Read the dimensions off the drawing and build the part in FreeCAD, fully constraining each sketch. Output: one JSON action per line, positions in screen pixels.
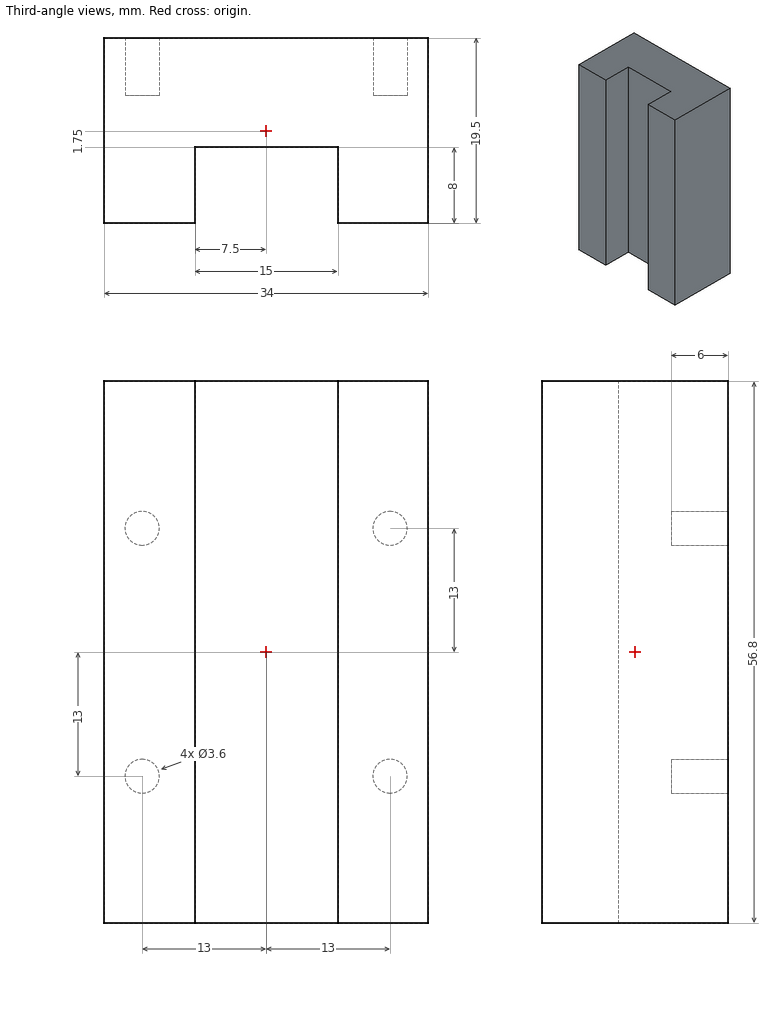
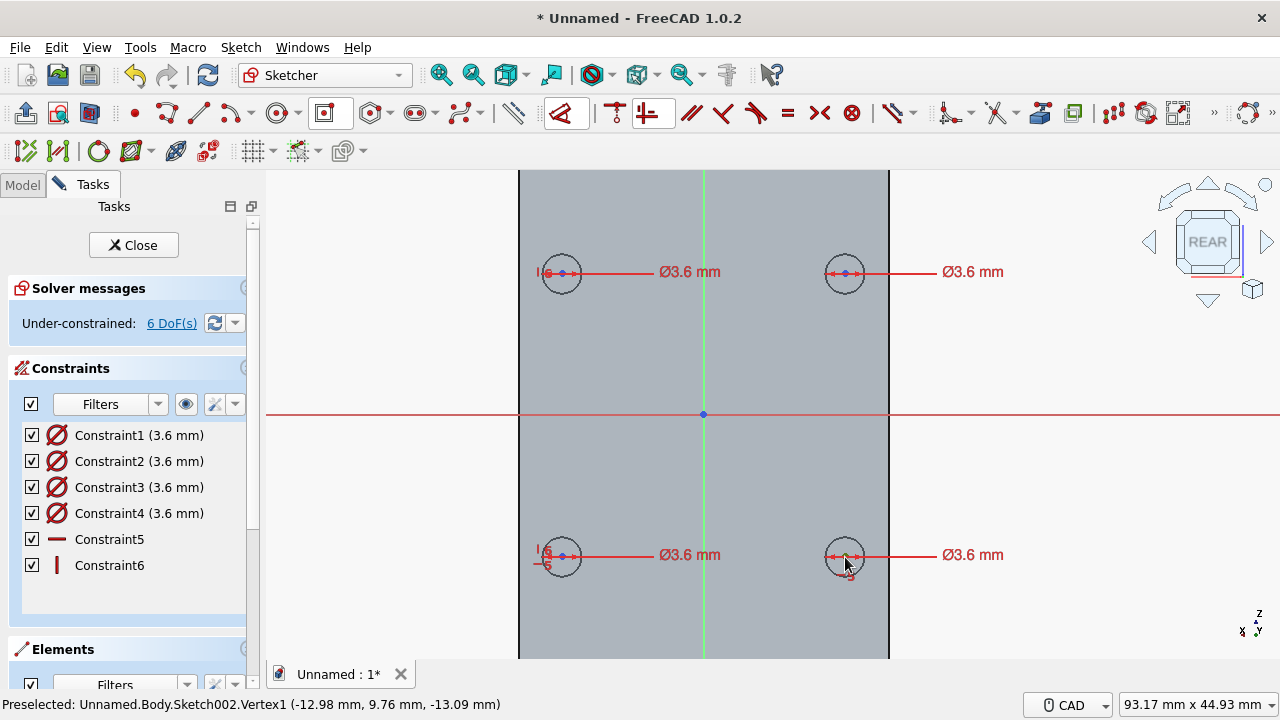
{"action": "left_click", "coordinate": [845, 274]}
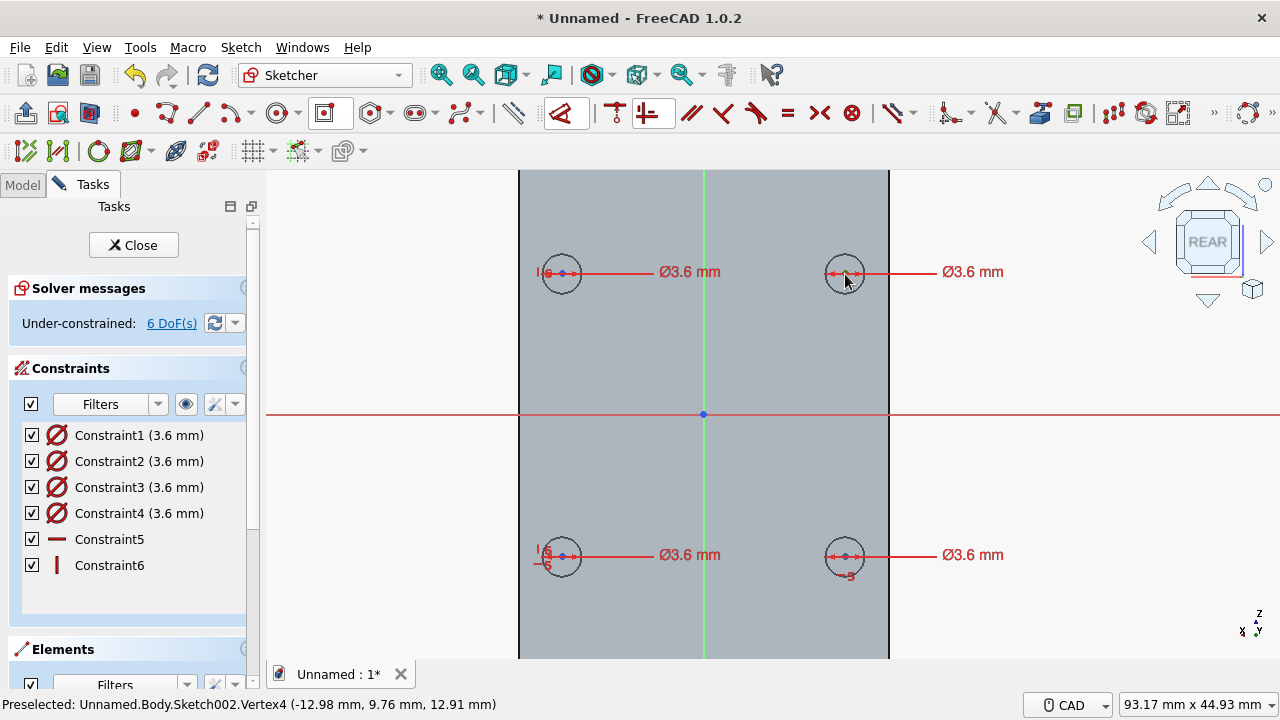
{"action": "key", "text": "v"}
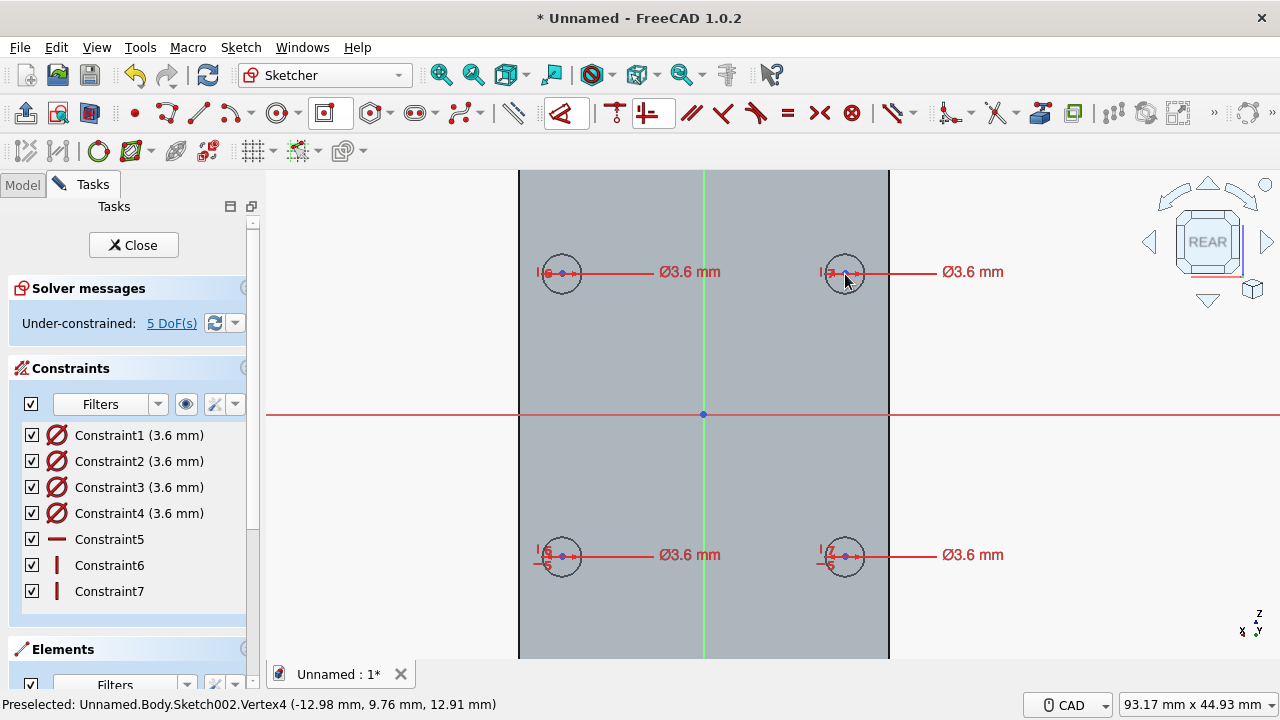
{"action": "left_click", "coordinate": [562, 274]}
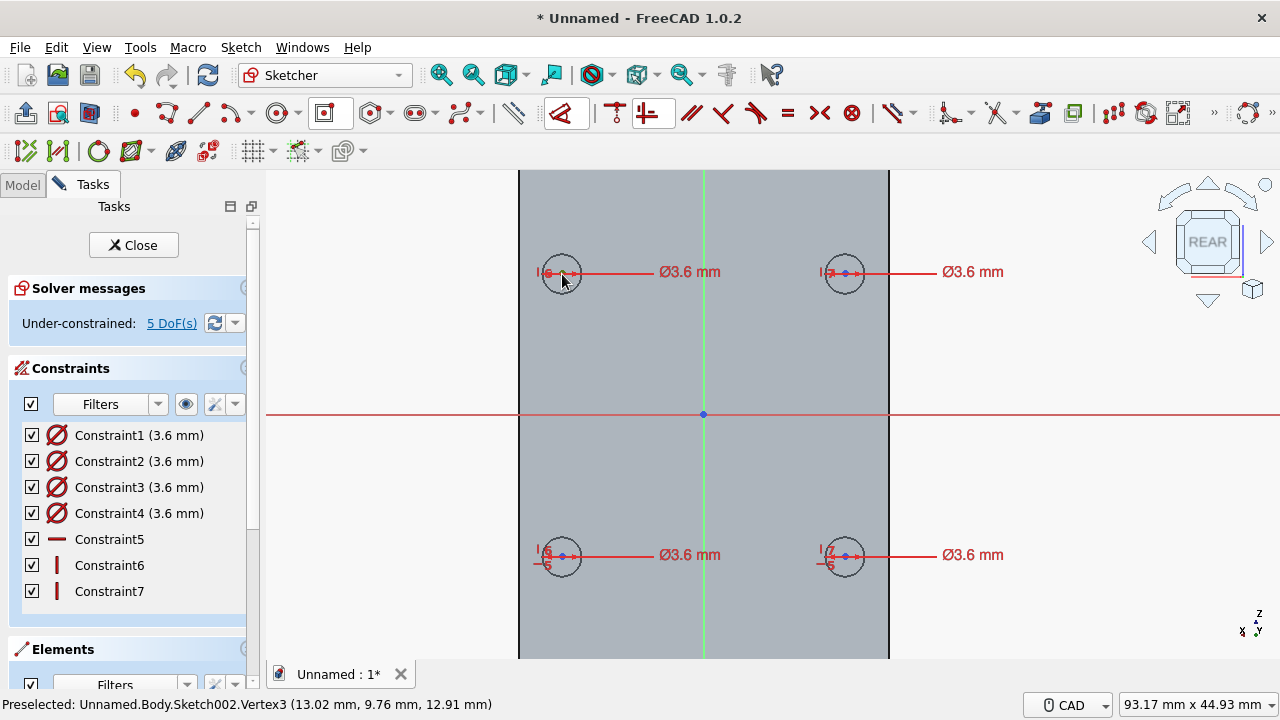
{"action": "left_click", "coordinate": [845, 274]}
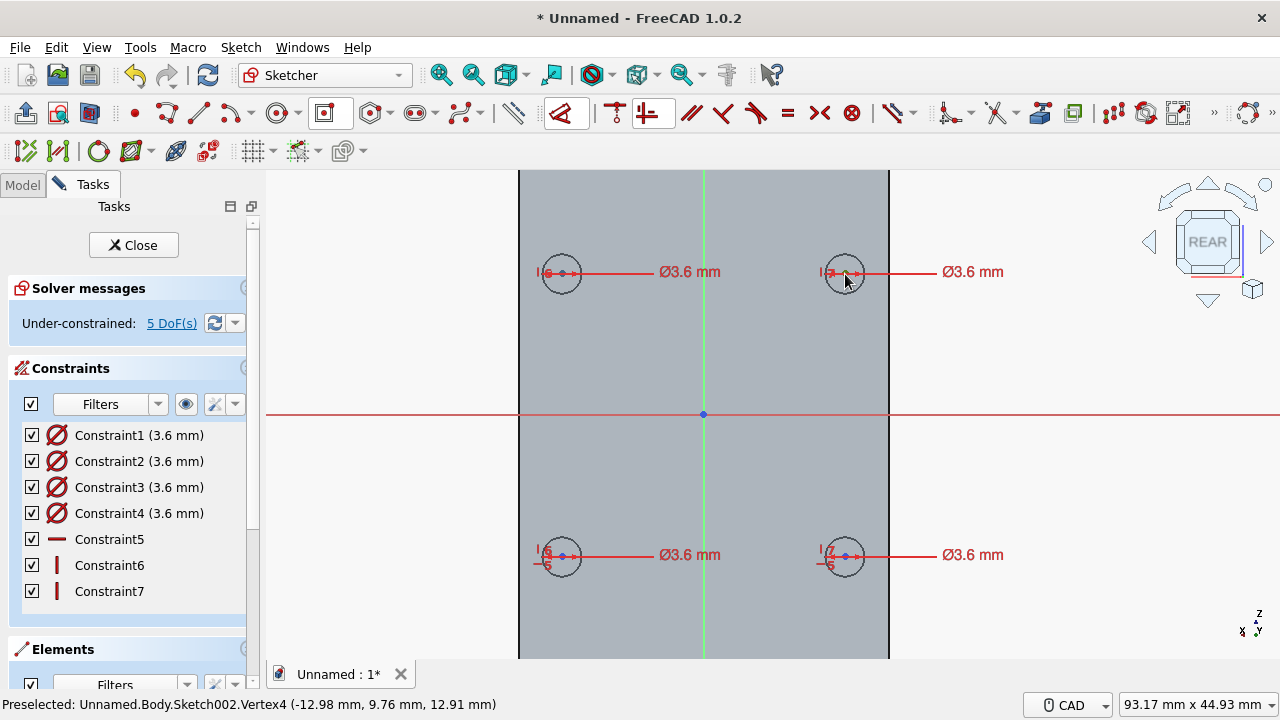
{"action": "left_click", "coordinate": [670, 114]}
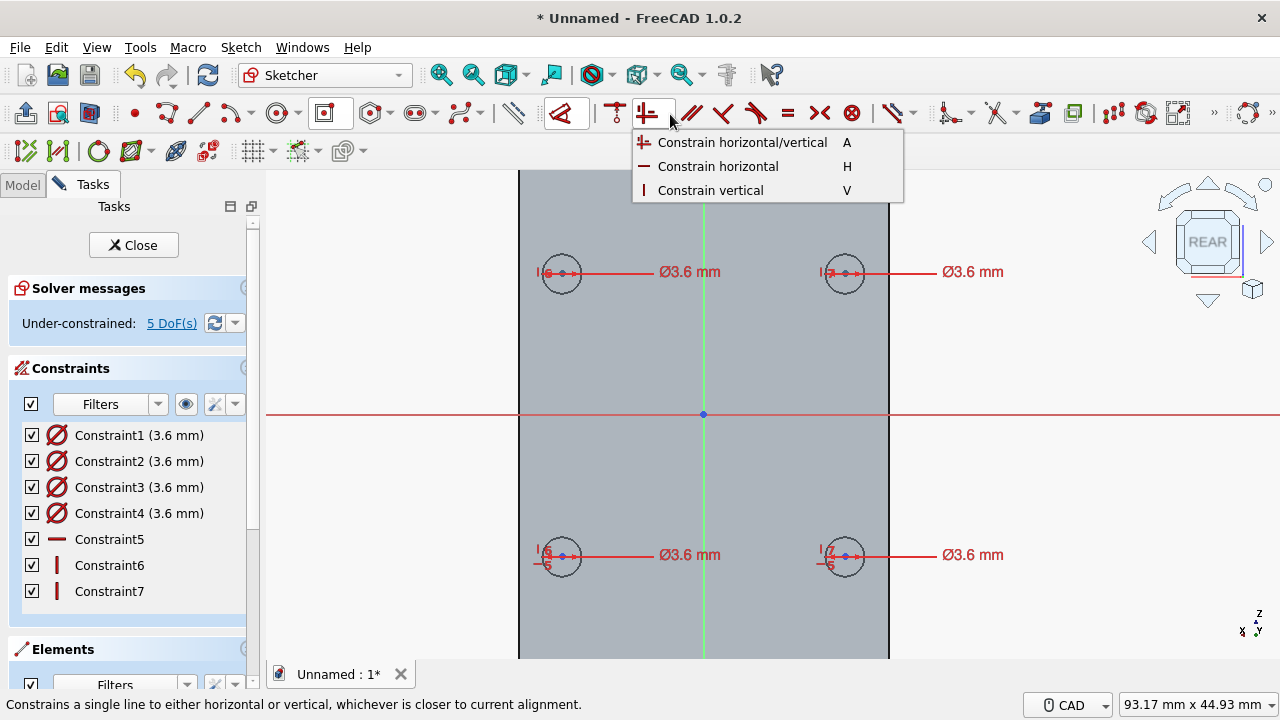
{"action": "left_click", "coordinate": [768, 166]}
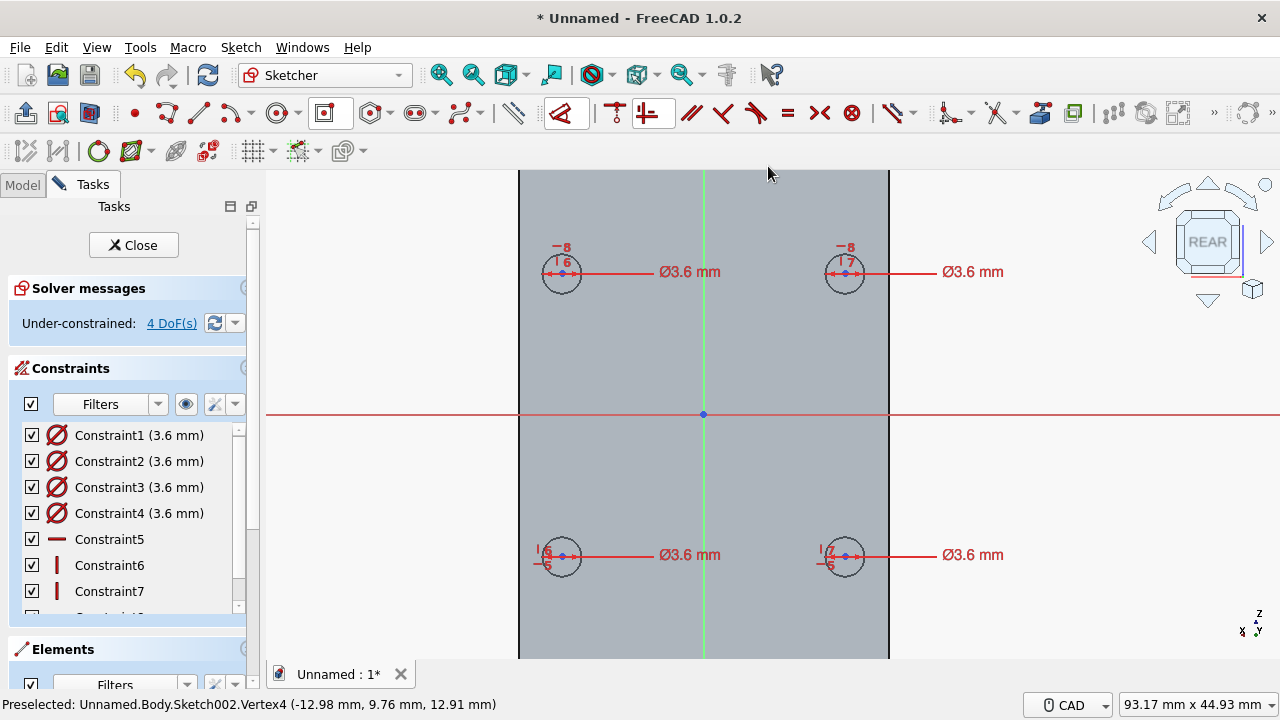
{"action": "left_click", "coordinate": [845, 557]}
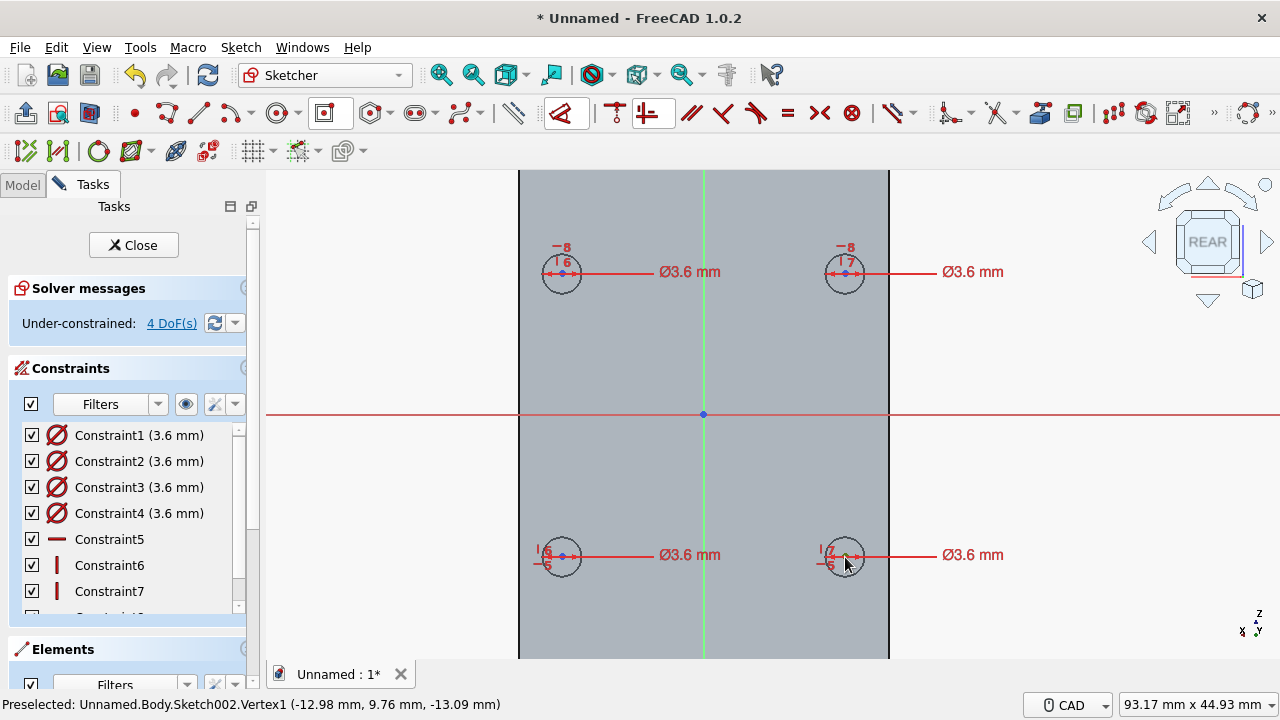
{"action": "key", "text": "l"}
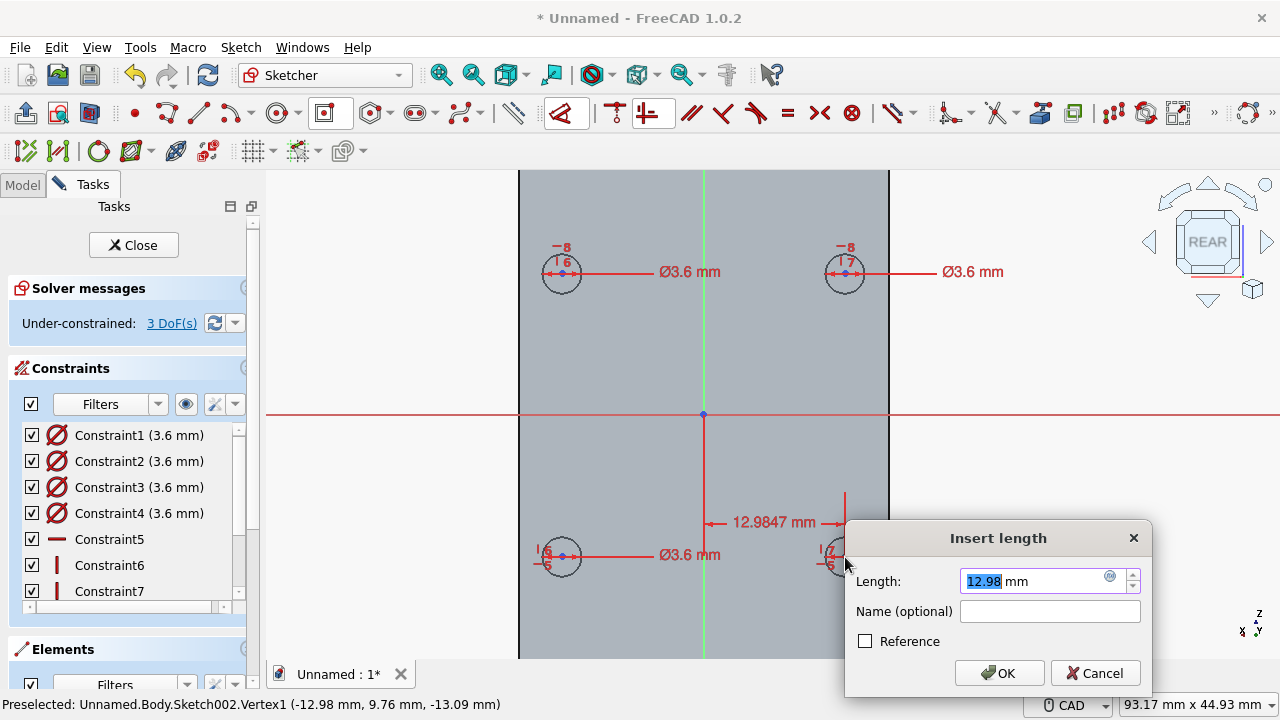
{"action": "type", "text": "13"}
{"action": "key", "text": "Return"}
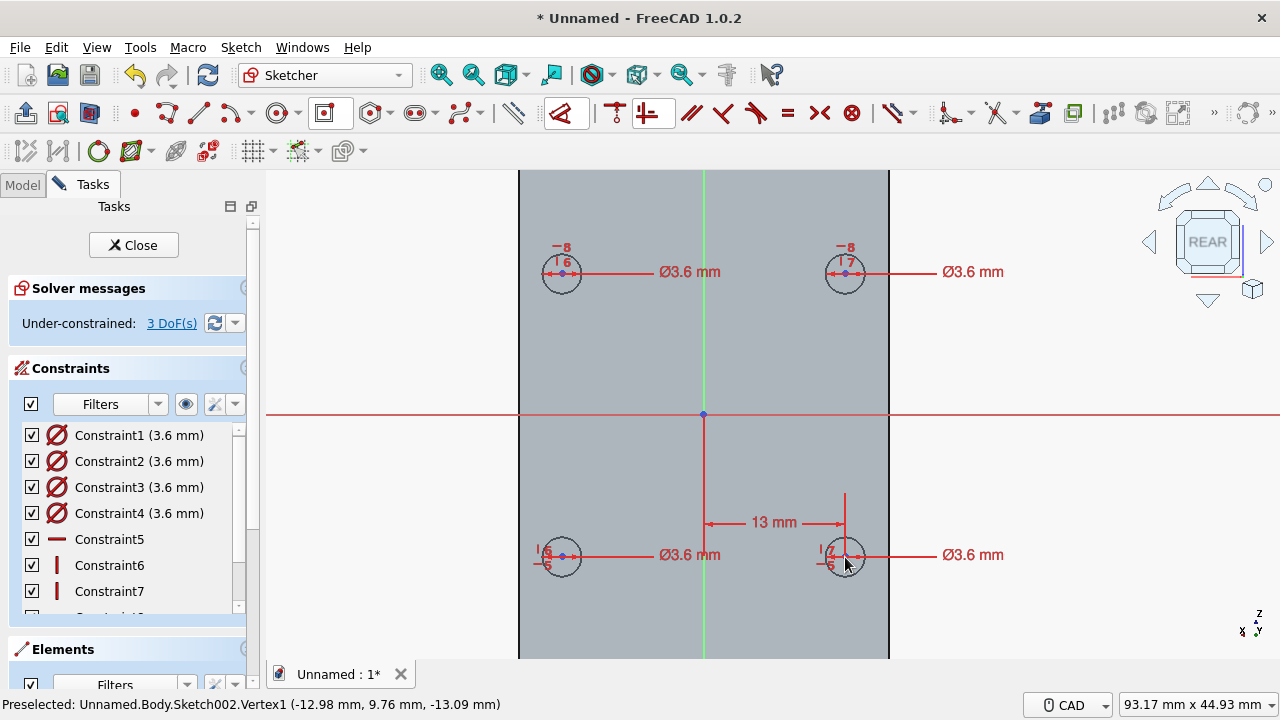
{"action": "left_click", "coordinate": [845, 557]}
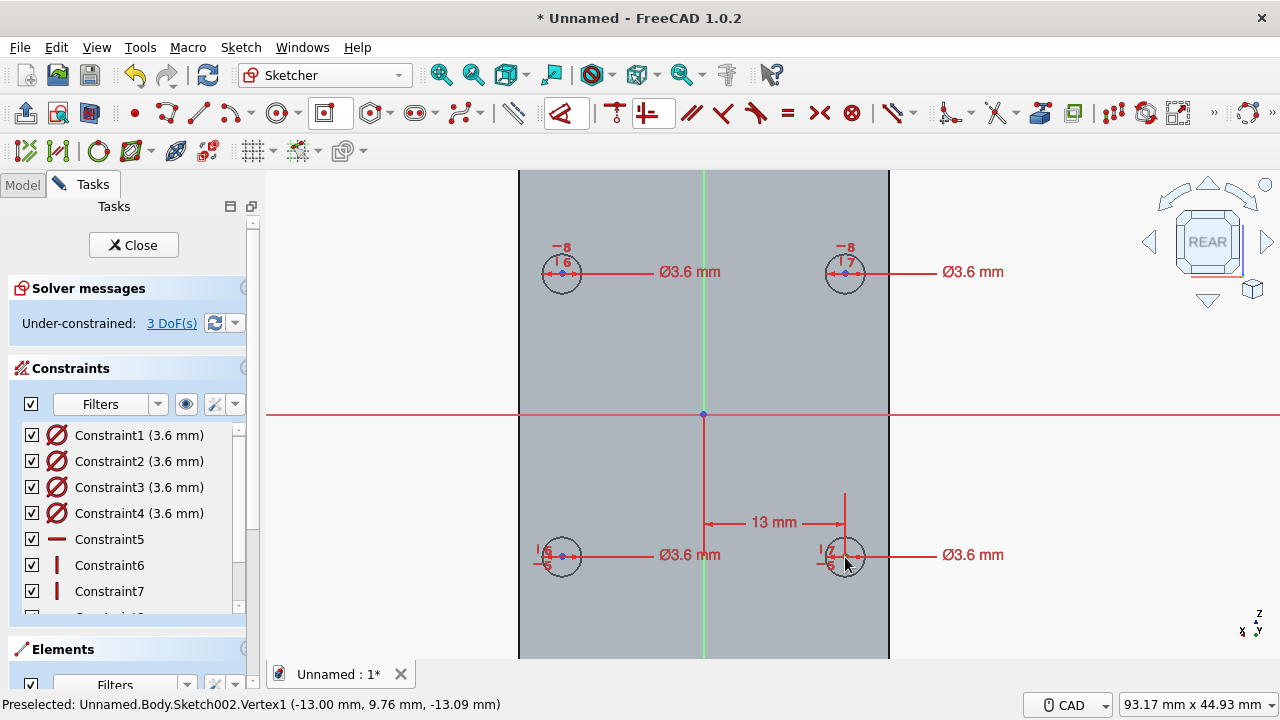
{"action": "left_click", "coordinate": [584, 114]}